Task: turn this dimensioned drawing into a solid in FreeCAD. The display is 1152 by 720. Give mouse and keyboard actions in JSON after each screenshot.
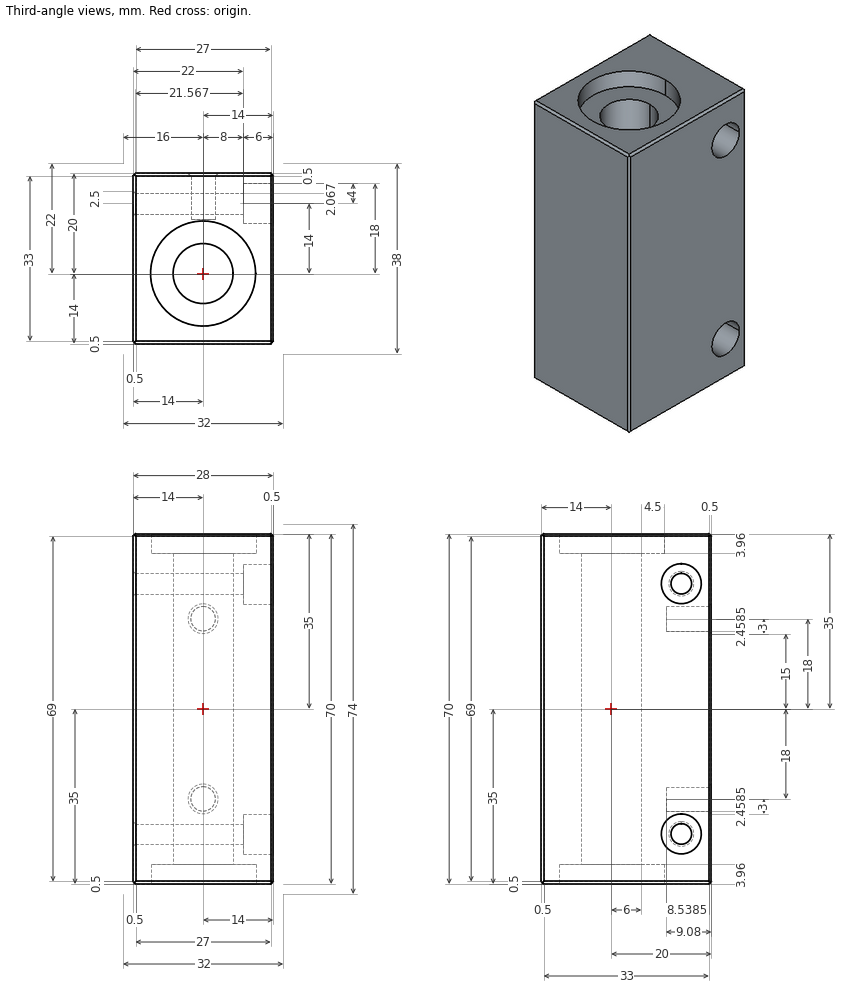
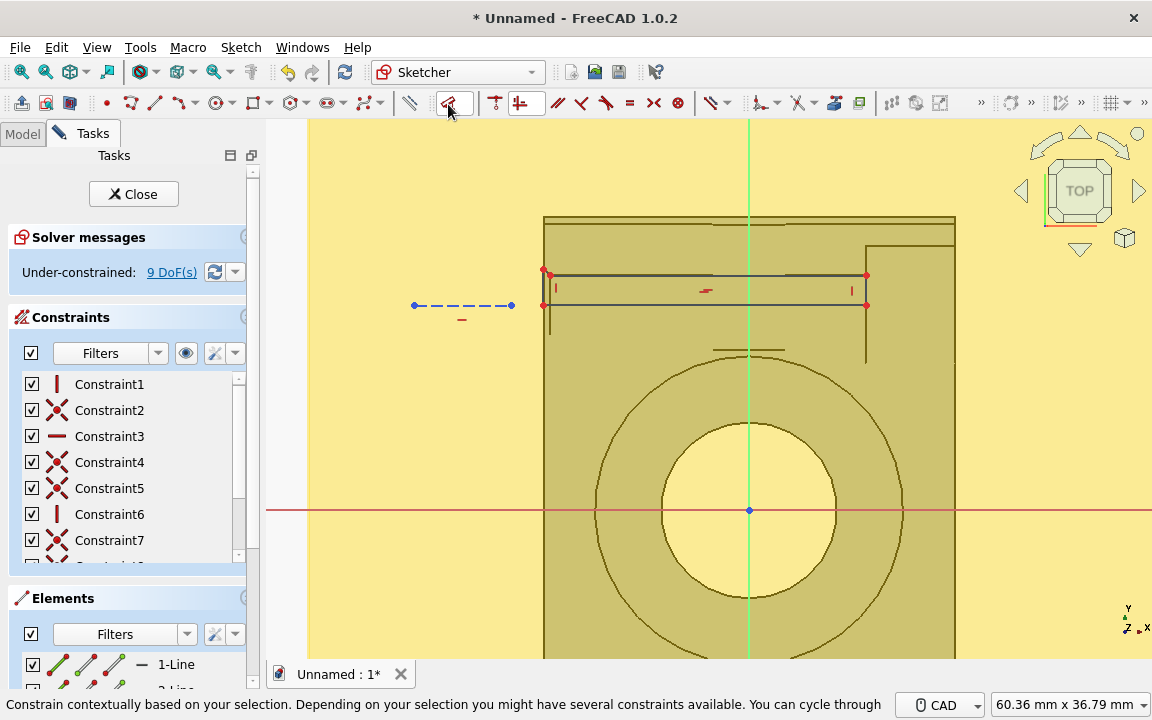
{"action": "left_click", "coordinate": [640, 305]}
{"action": "left_click", "coordinate": [705, 339]}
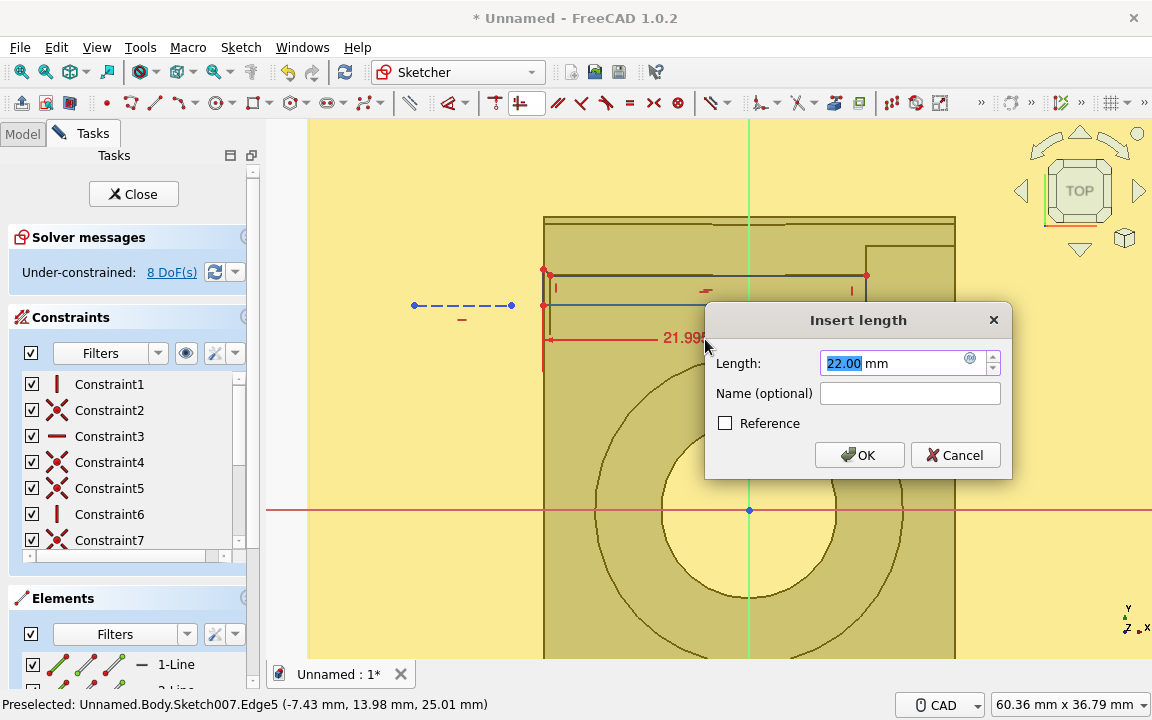
{"action": "type", "text": "22"}
{"action": "key", "text": "Return"}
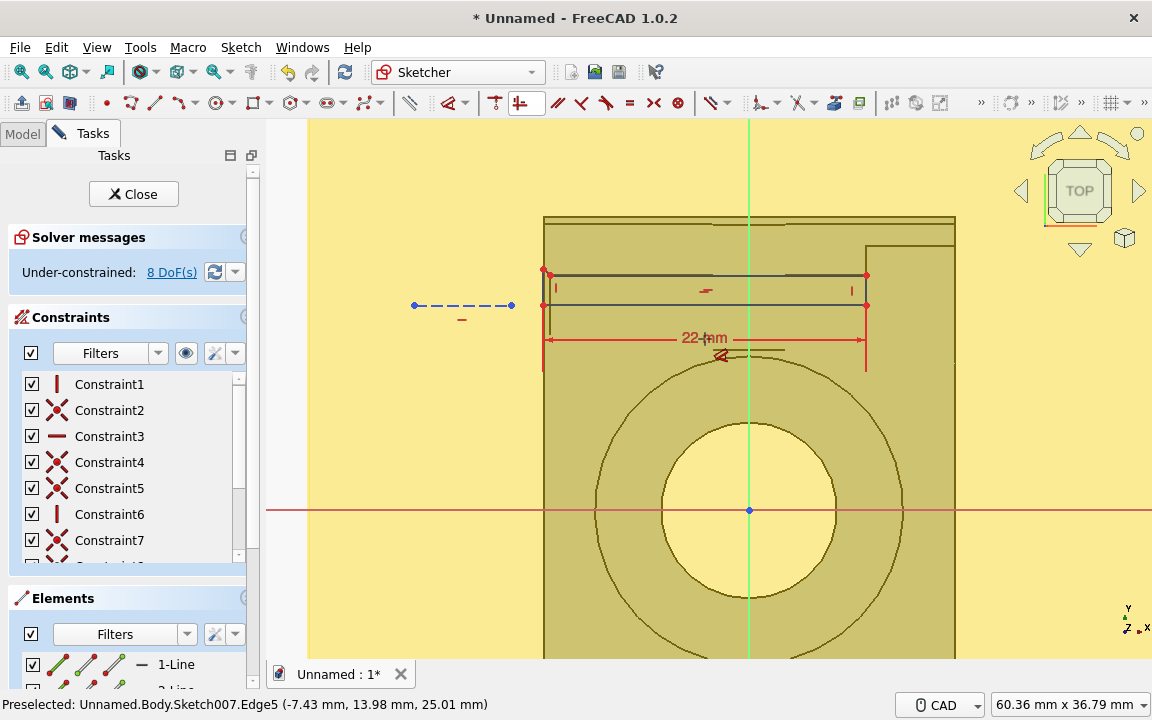
{"action": "left_click", "coordinate": [866, 305]}
{"action": "left_click", "coordinate": [808, 544]}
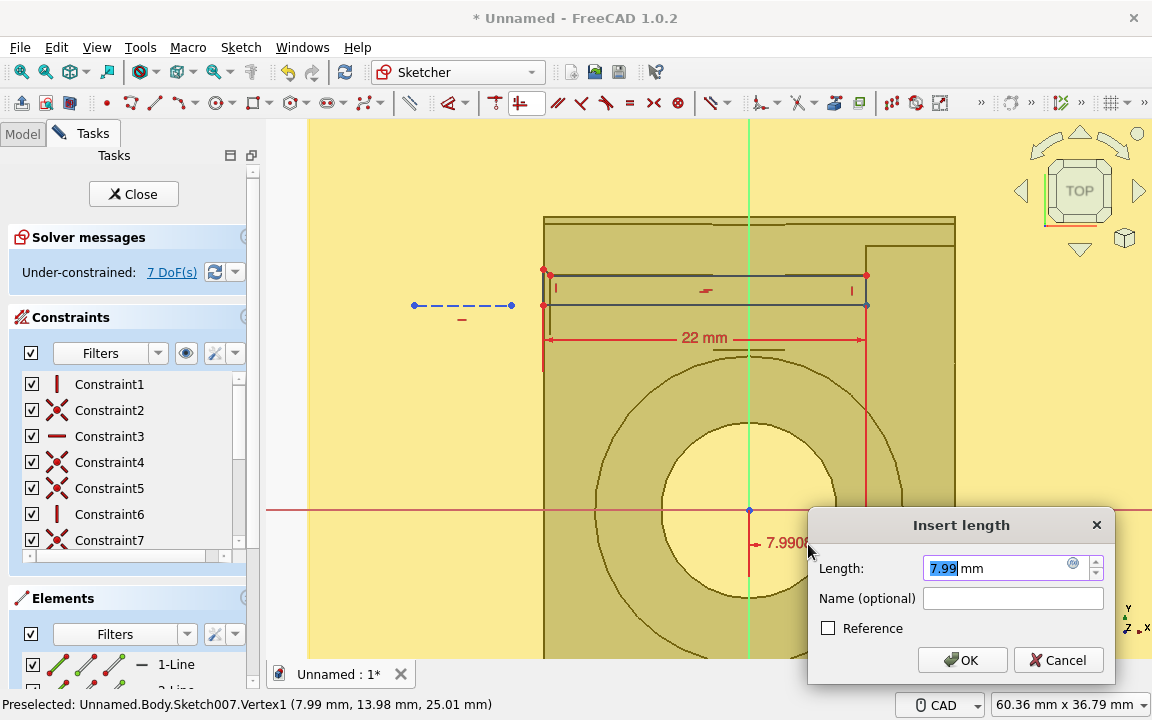
{"action": "type", "text": "8"}
{"action": "key", "text": "Return"}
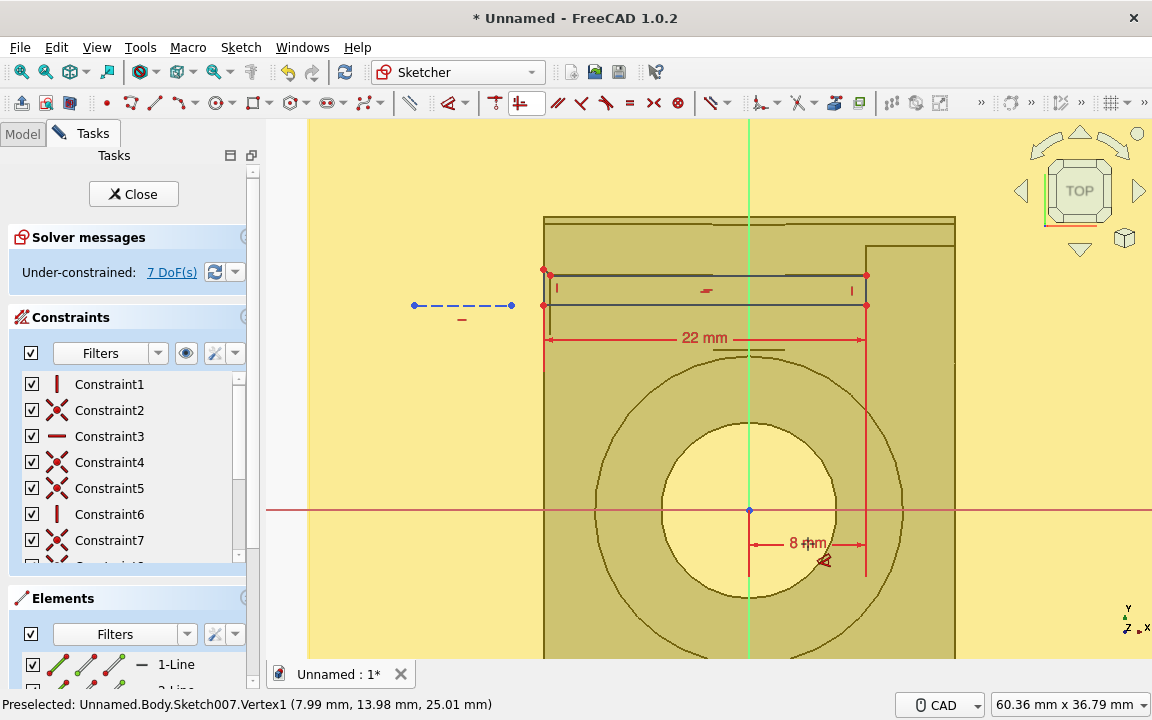
{"action": "scroll", "coordinate": [544, 294], "scroll_direction": "up", "scroll_amount": 2}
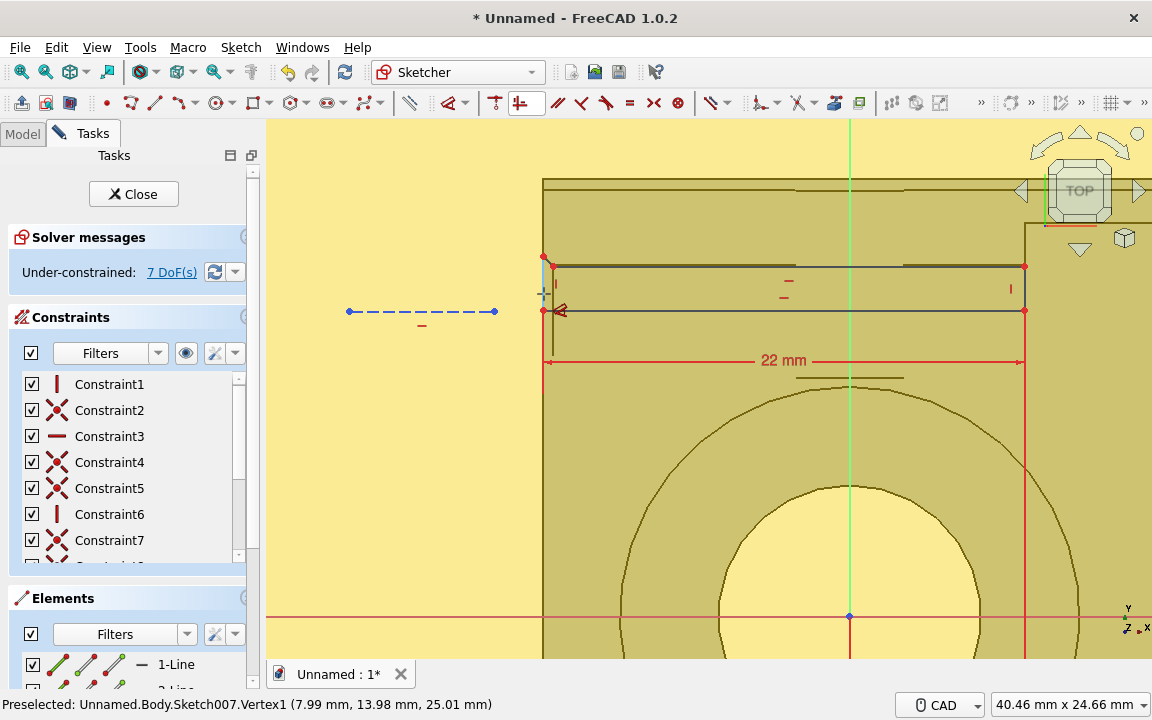
{"action": "left_click", "coordinate": [543, 294]}
{"action": "left_click", "coordinate": [509, 284]}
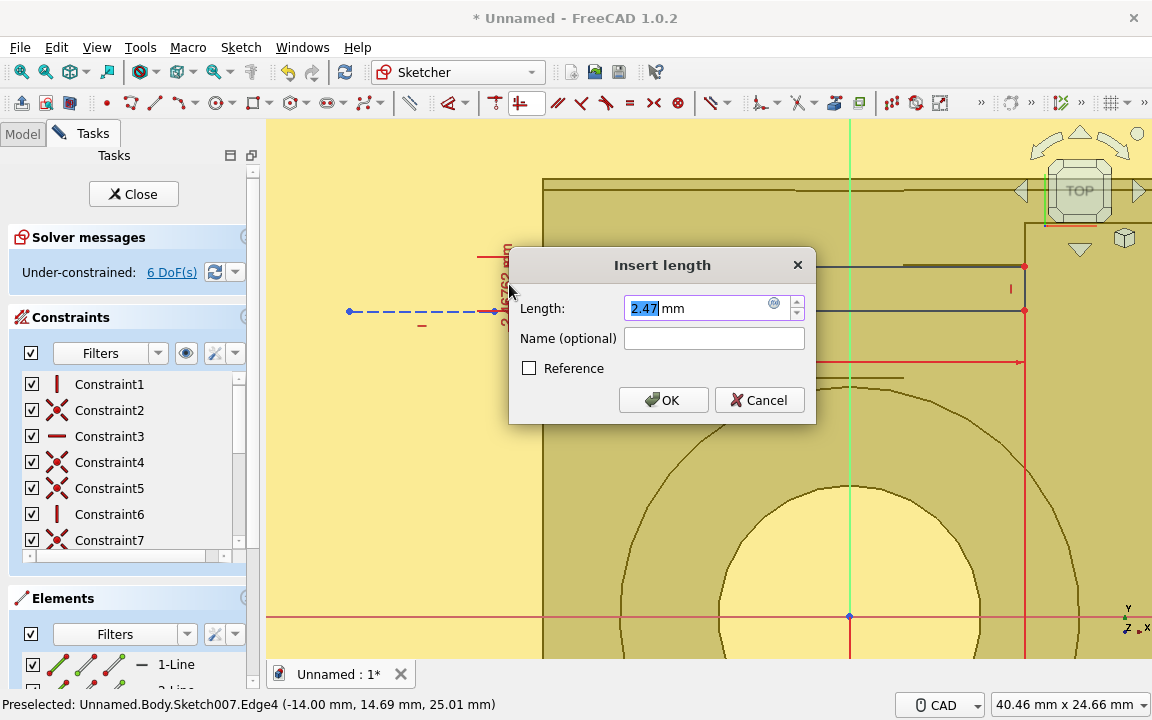
{"action": "type", "text": "2.5"}
{"action": "key", "text": "Return"}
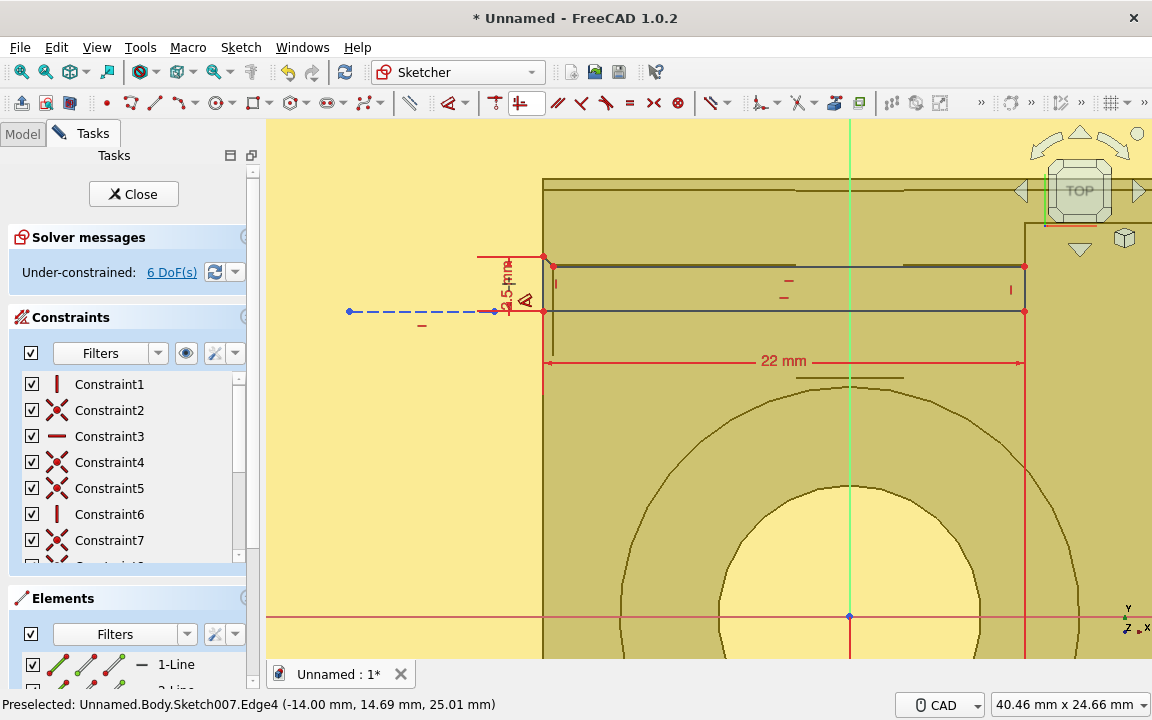
{"action": "scroll", "coordinate": [545, 293], "scroll_direction": "down", "scroll_amount": 2}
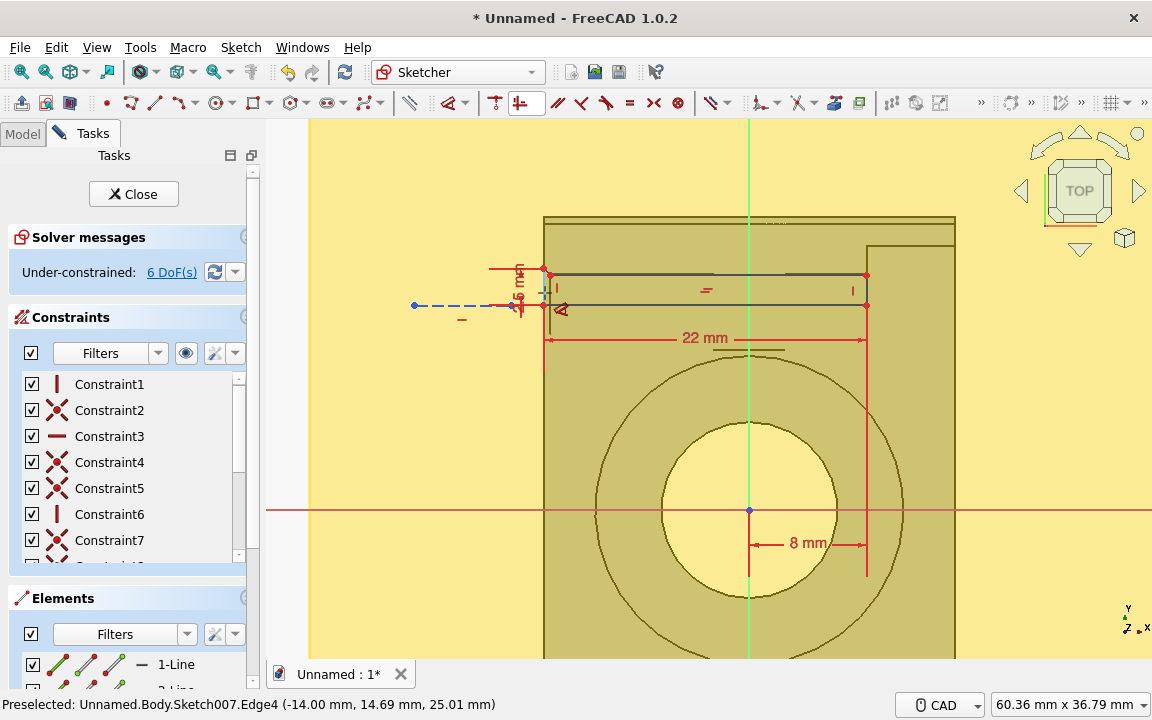
{"action": "left_click", "coordinate": [867, 305]}
{"action": "left_click", "coordinate": [901, 408]}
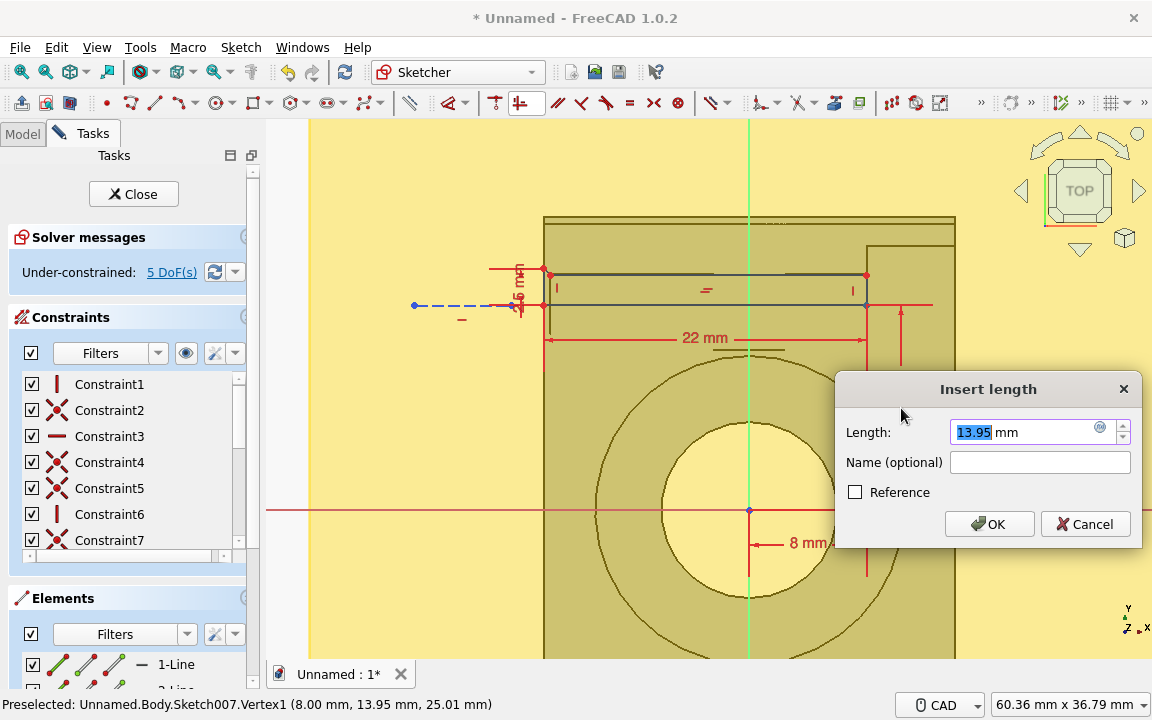
{"action": "type", "text": "14"}
{"action": "key", "text": "Return"}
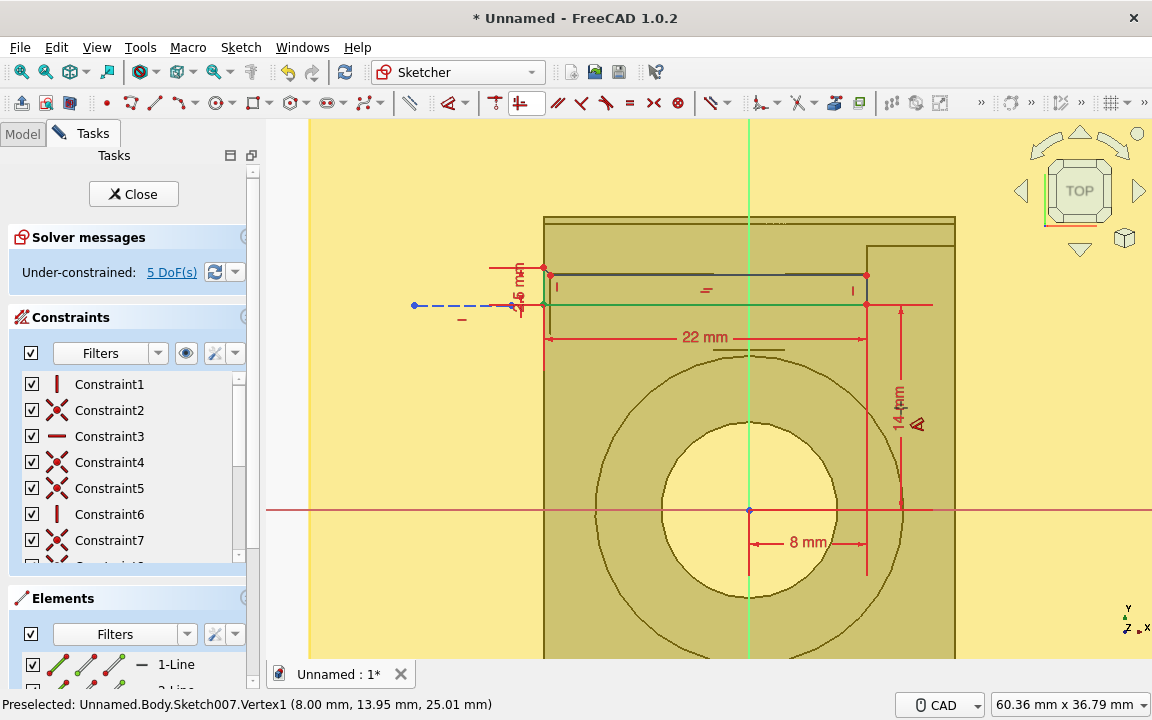
{"action": "left_click", "coordinate": [511, 306]}
{"action": "left_click", "coordinate": [477, 408]}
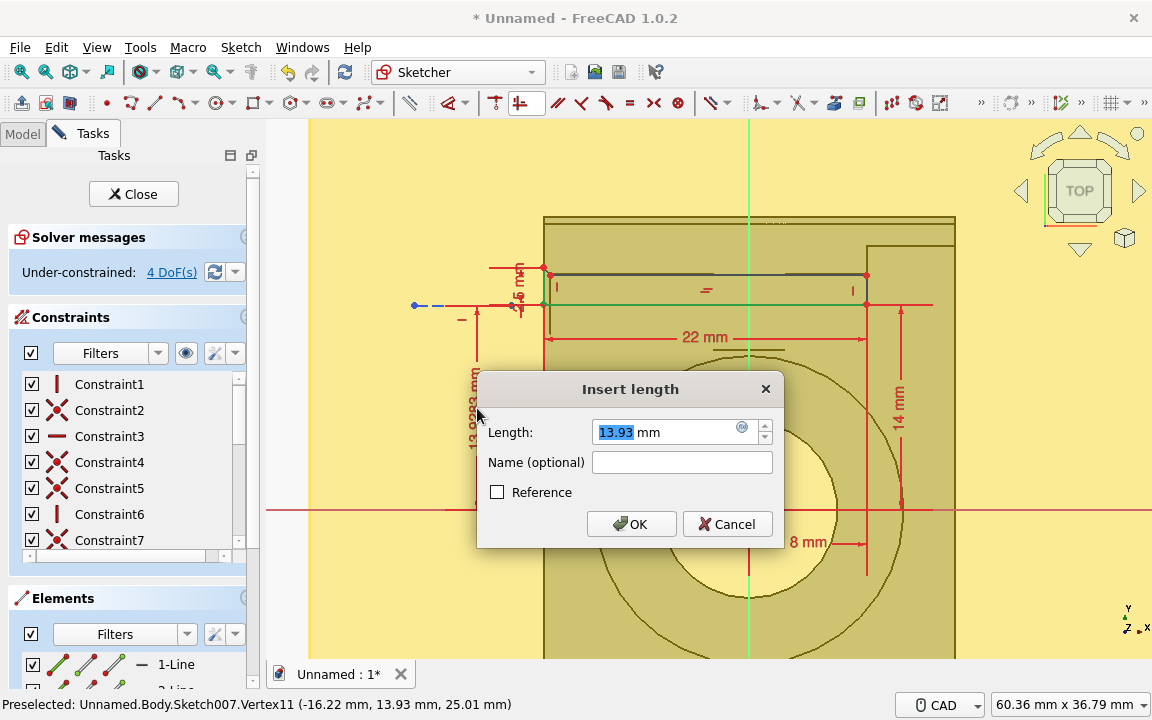
{"action": "type", "text": "14"}
{"action": "key", "text": "Return"}